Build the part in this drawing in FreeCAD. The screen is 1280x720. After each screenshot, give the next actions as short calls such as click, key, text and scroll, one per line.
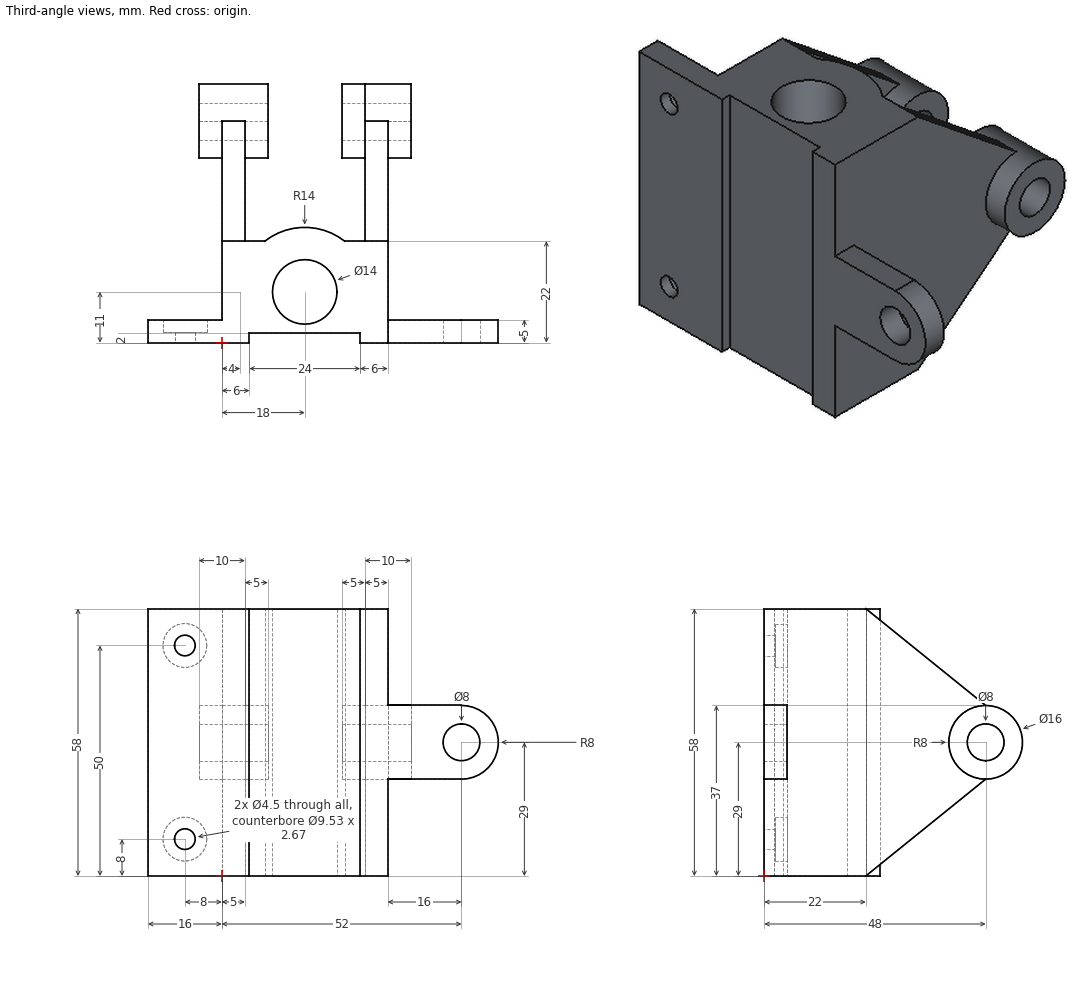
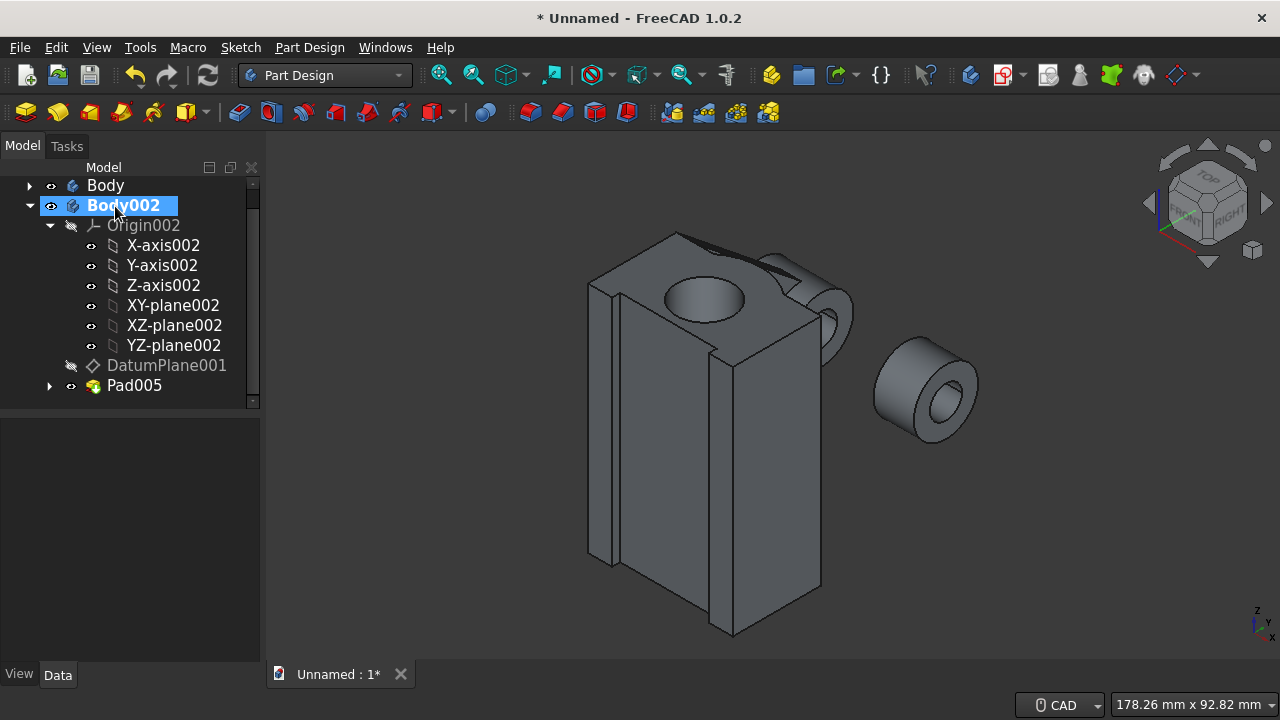
double_click(96, 186)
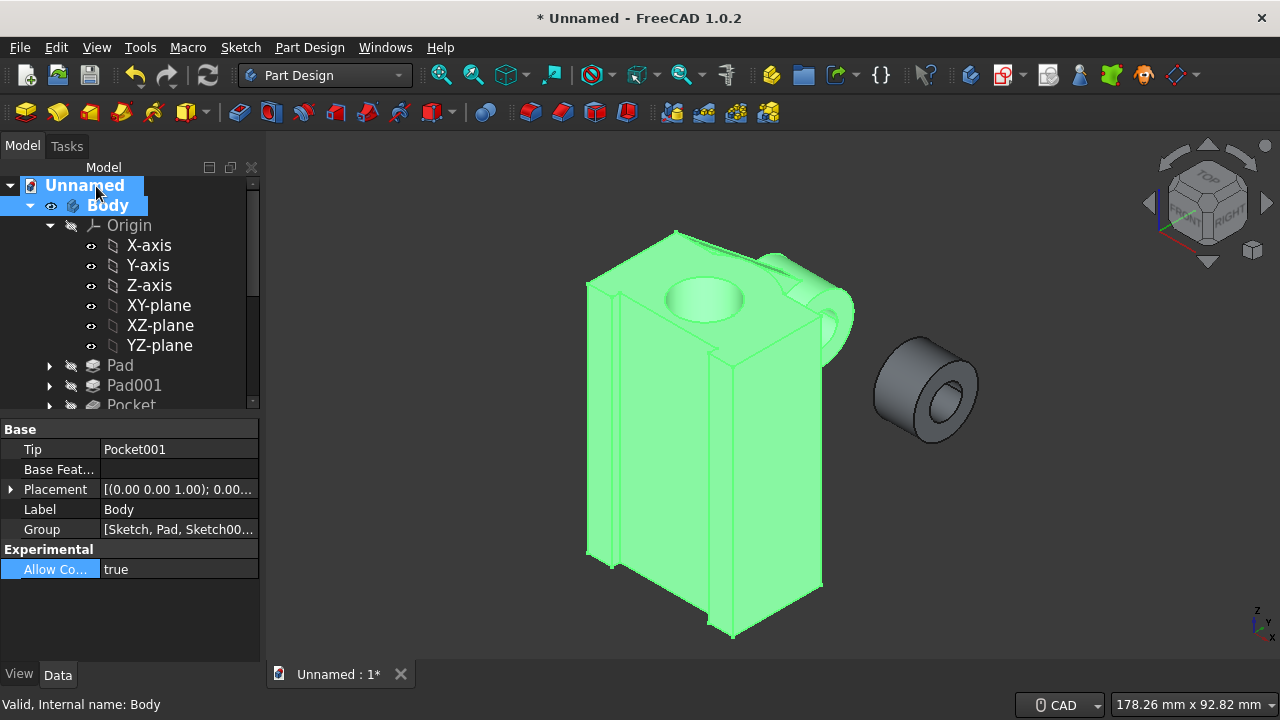
scroll(100, 301, down, 3)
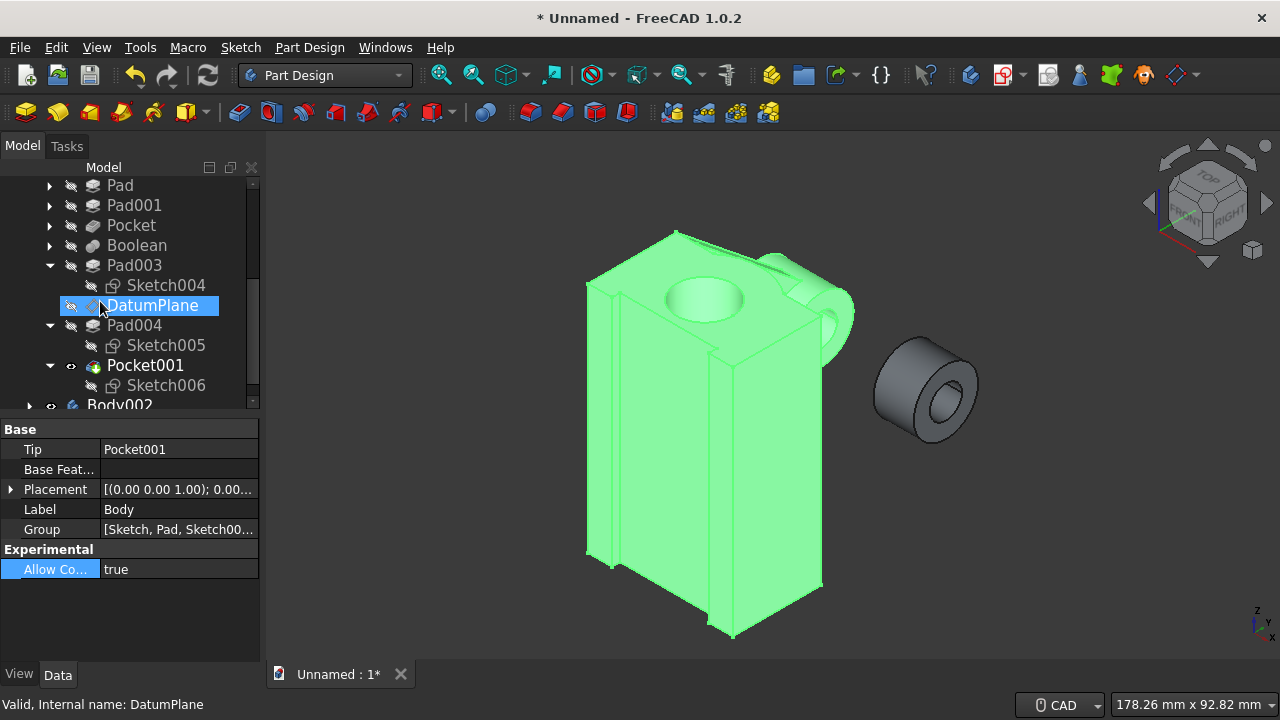
click(96, 406)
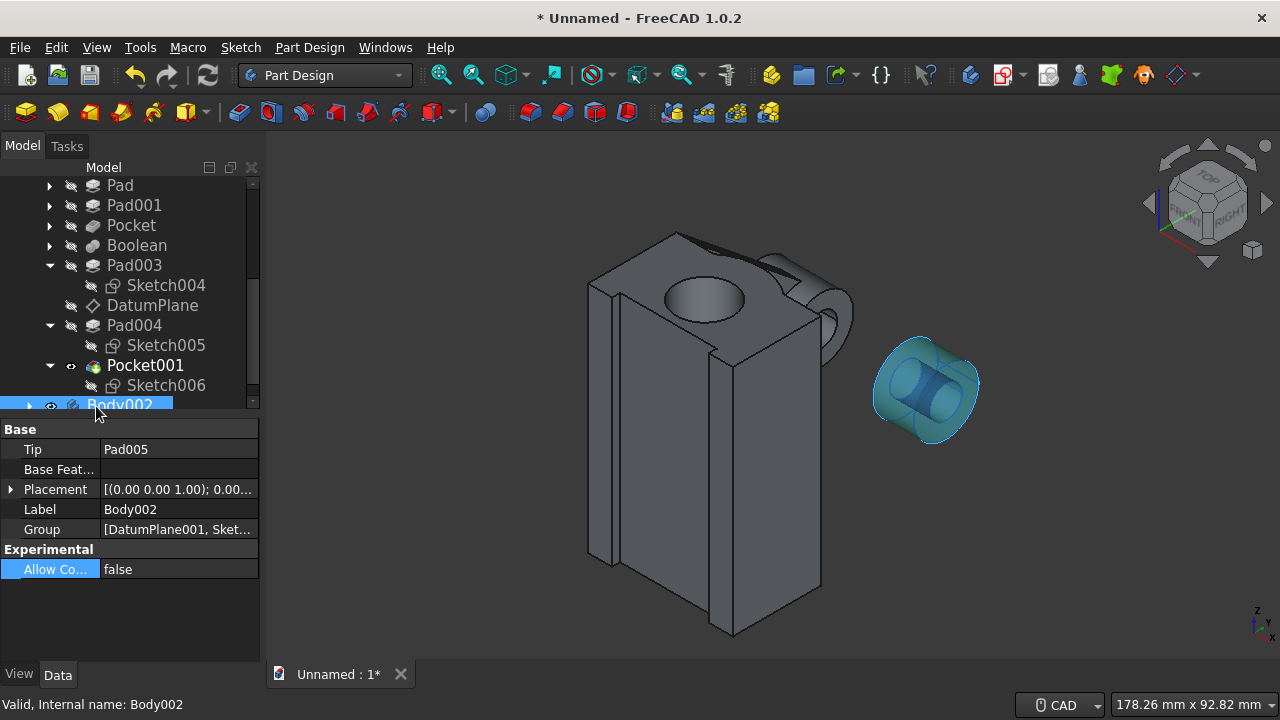
click(486, 112)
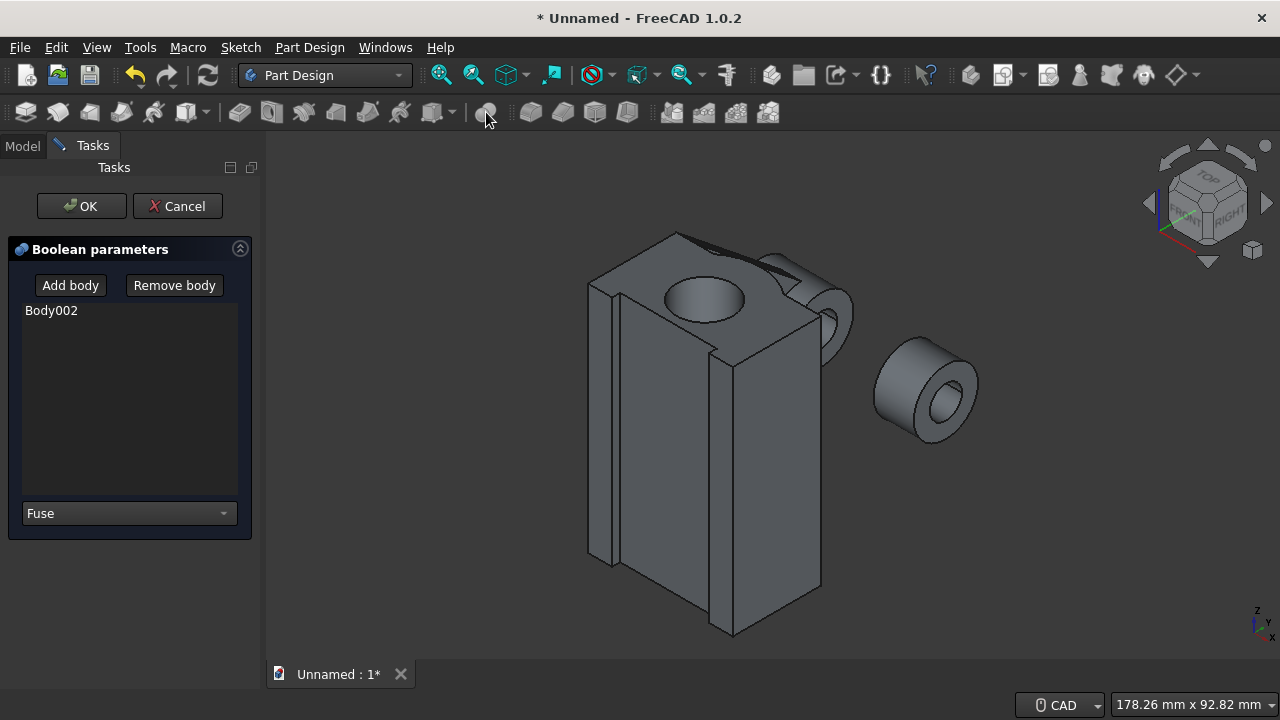
click(82, 206)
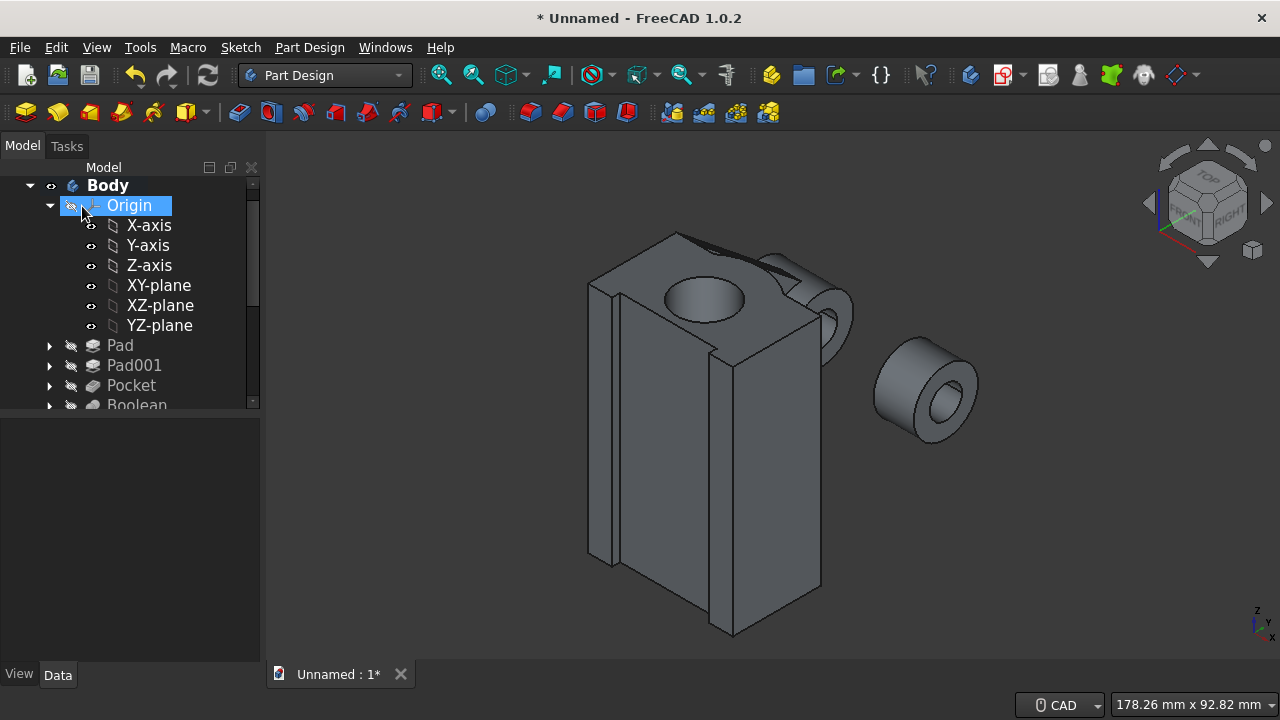
click(777, 398)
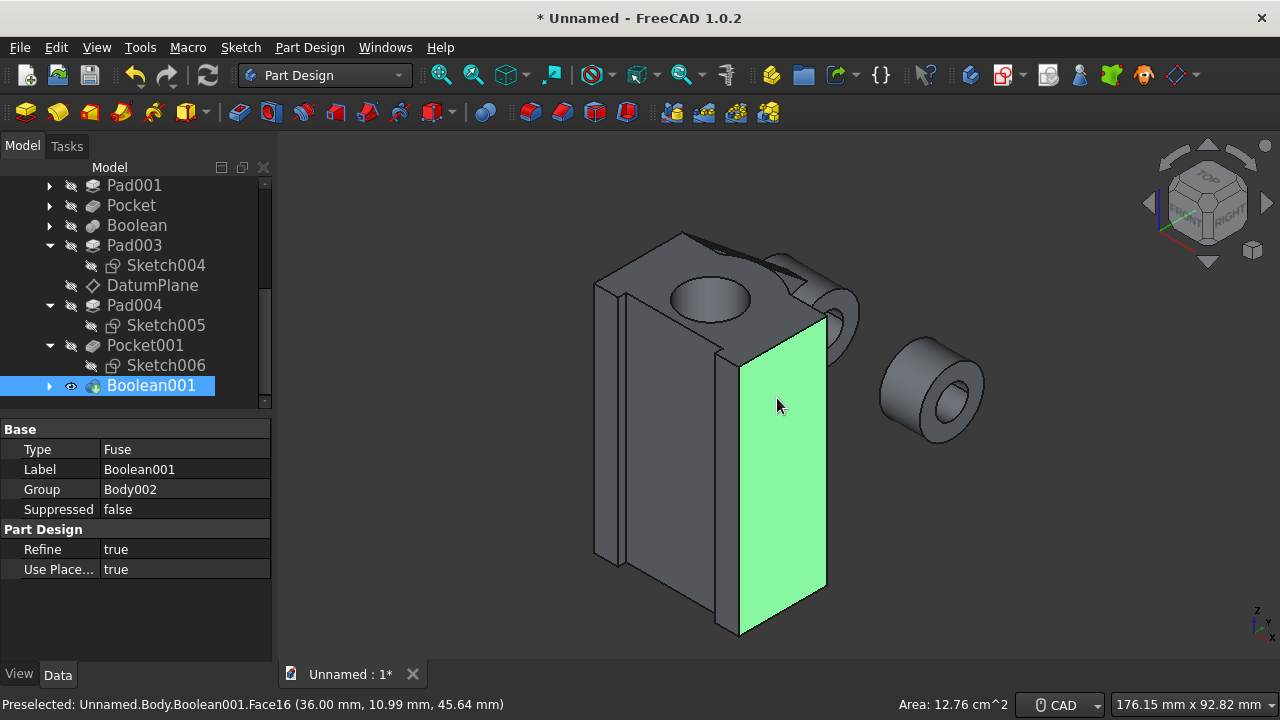
click(1004, 76)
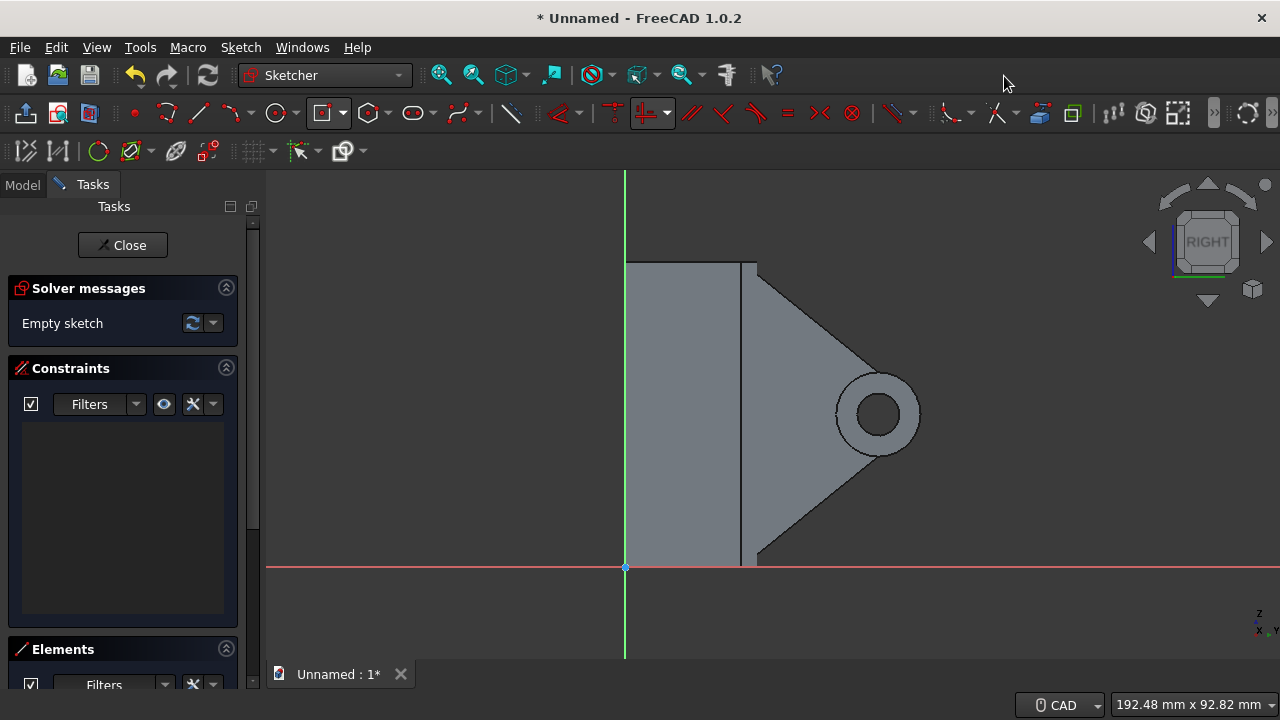
key(q)
key(s)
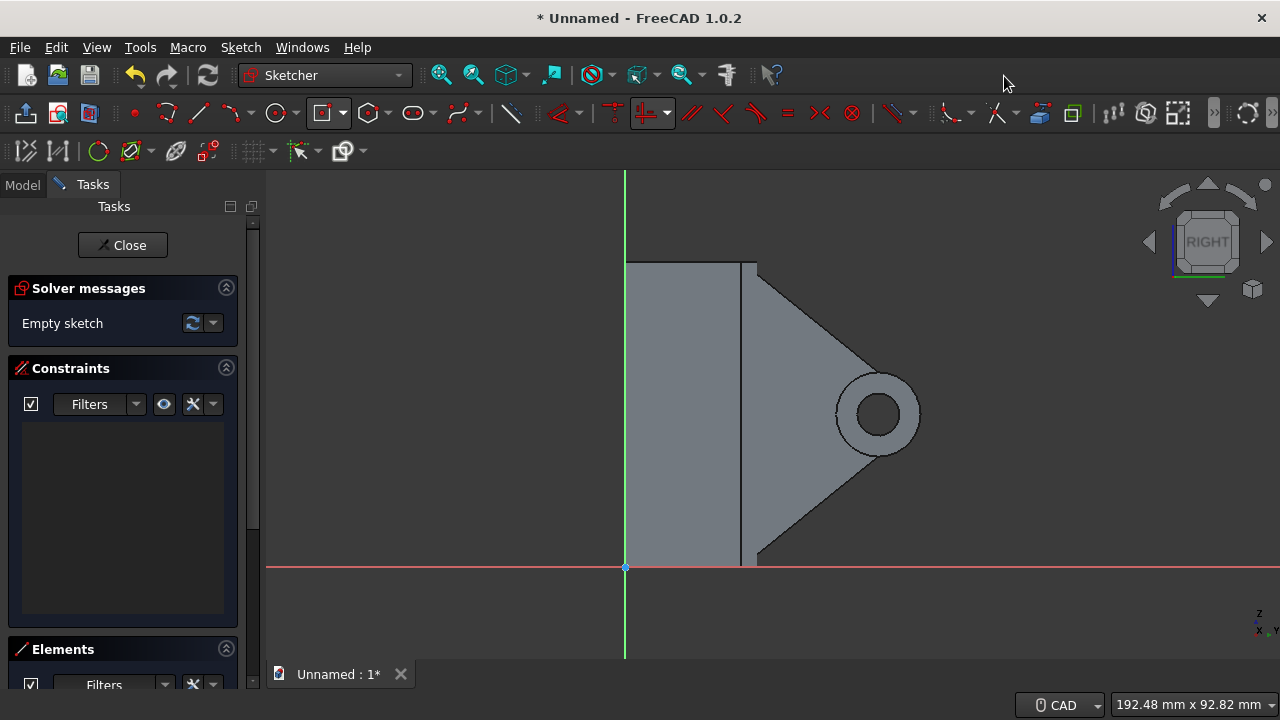
key(g)
key(m)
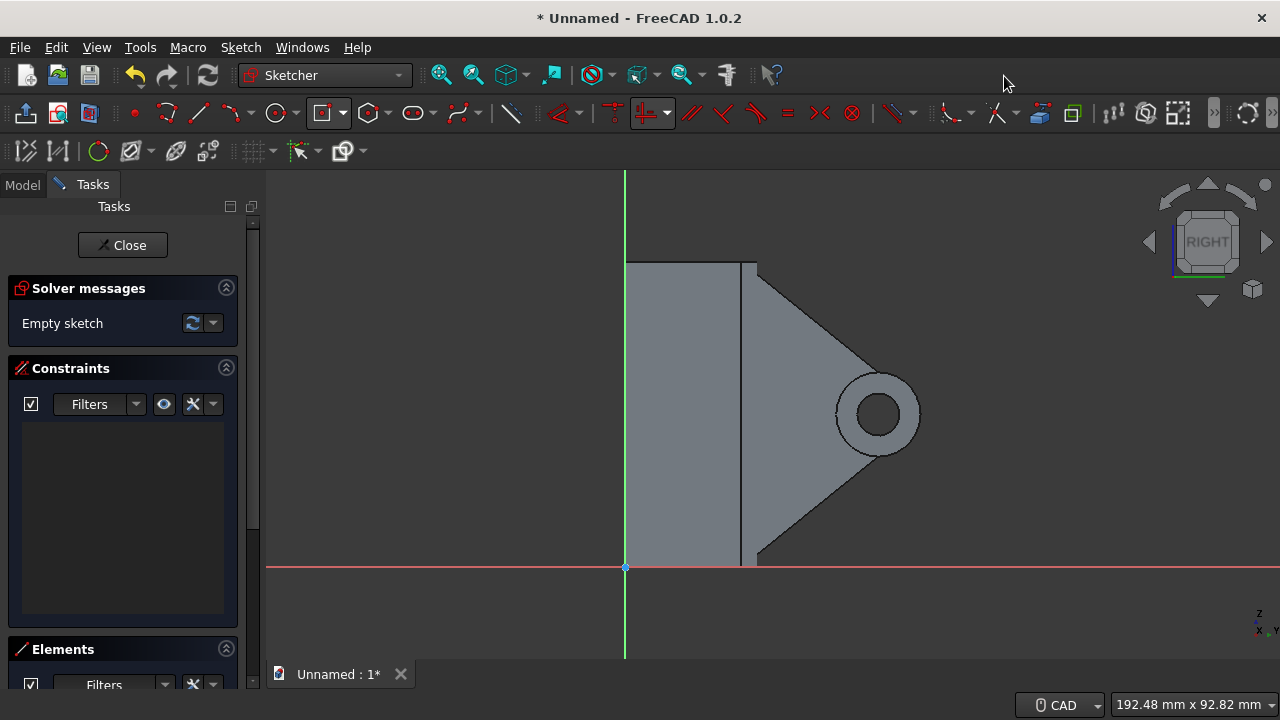
click(878, 372)
click(741, 262)
click(741, 567)
click(878, 457)
right_click(878, 457)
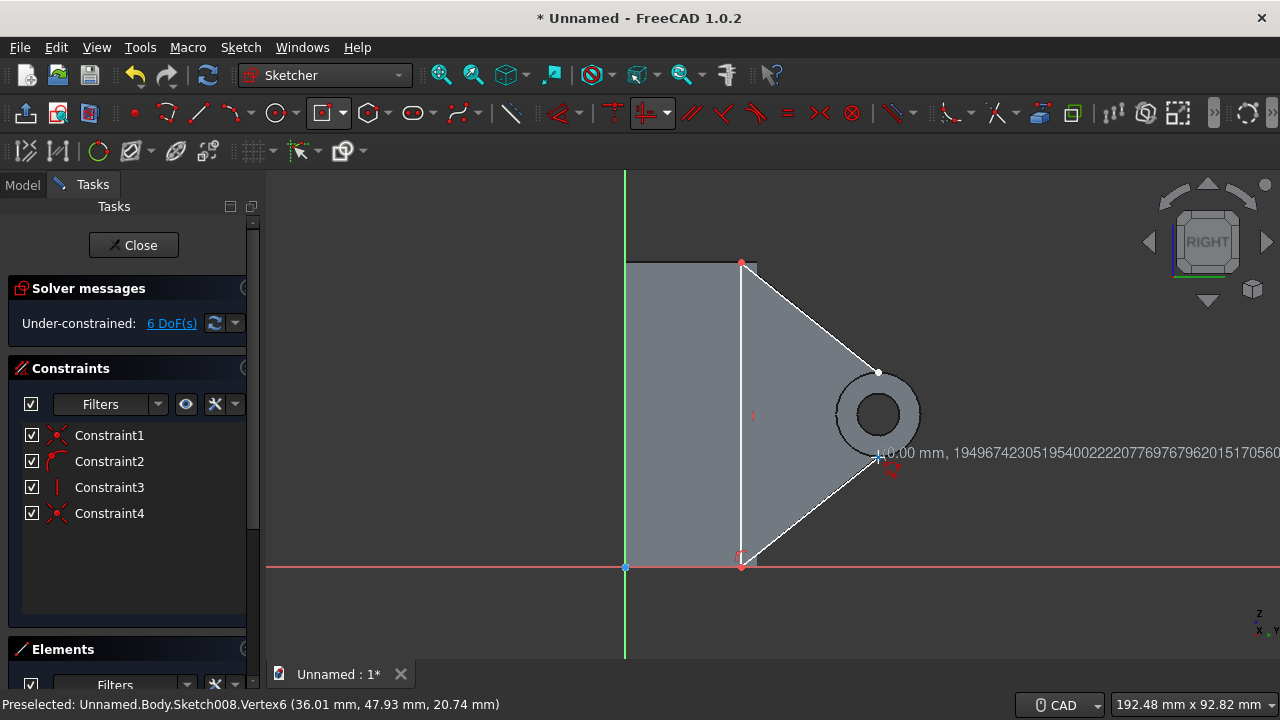
key(g)
key(3)
key(a)